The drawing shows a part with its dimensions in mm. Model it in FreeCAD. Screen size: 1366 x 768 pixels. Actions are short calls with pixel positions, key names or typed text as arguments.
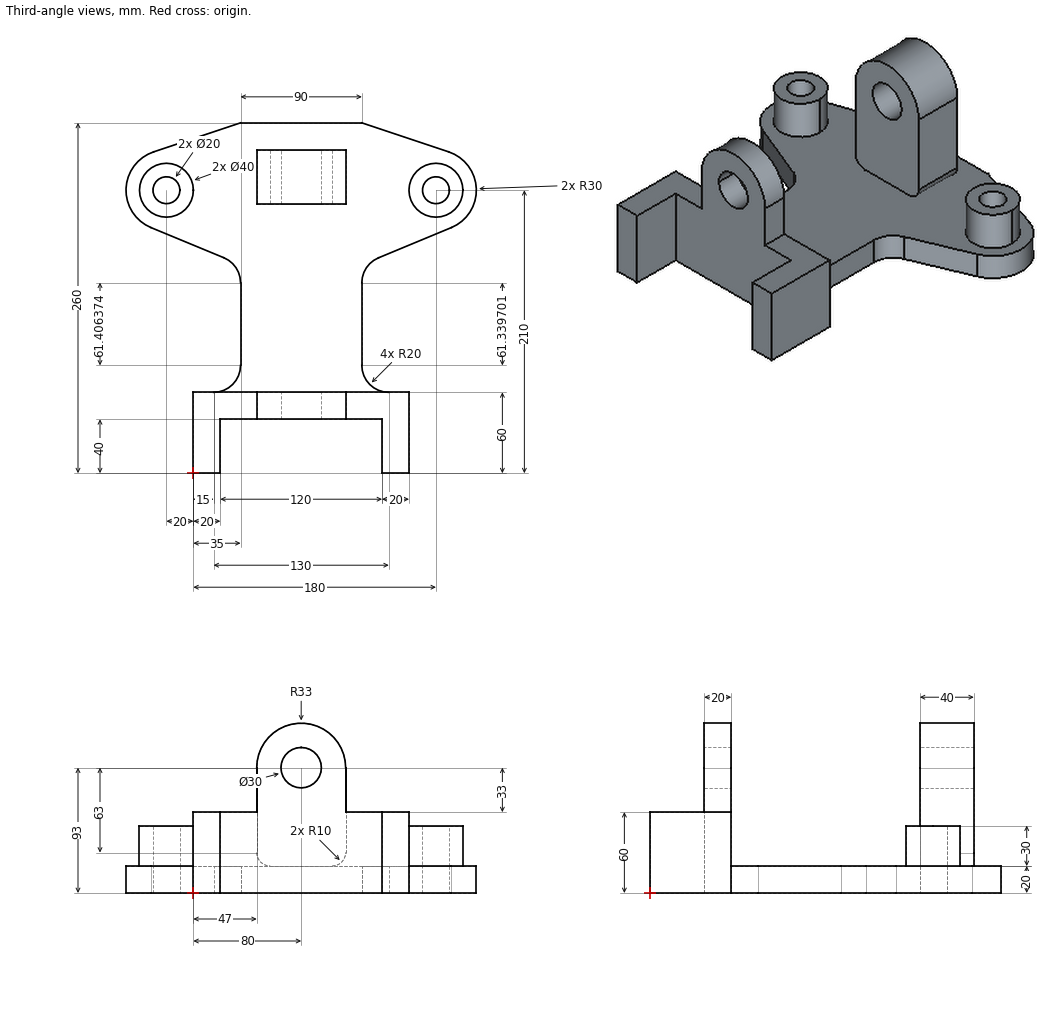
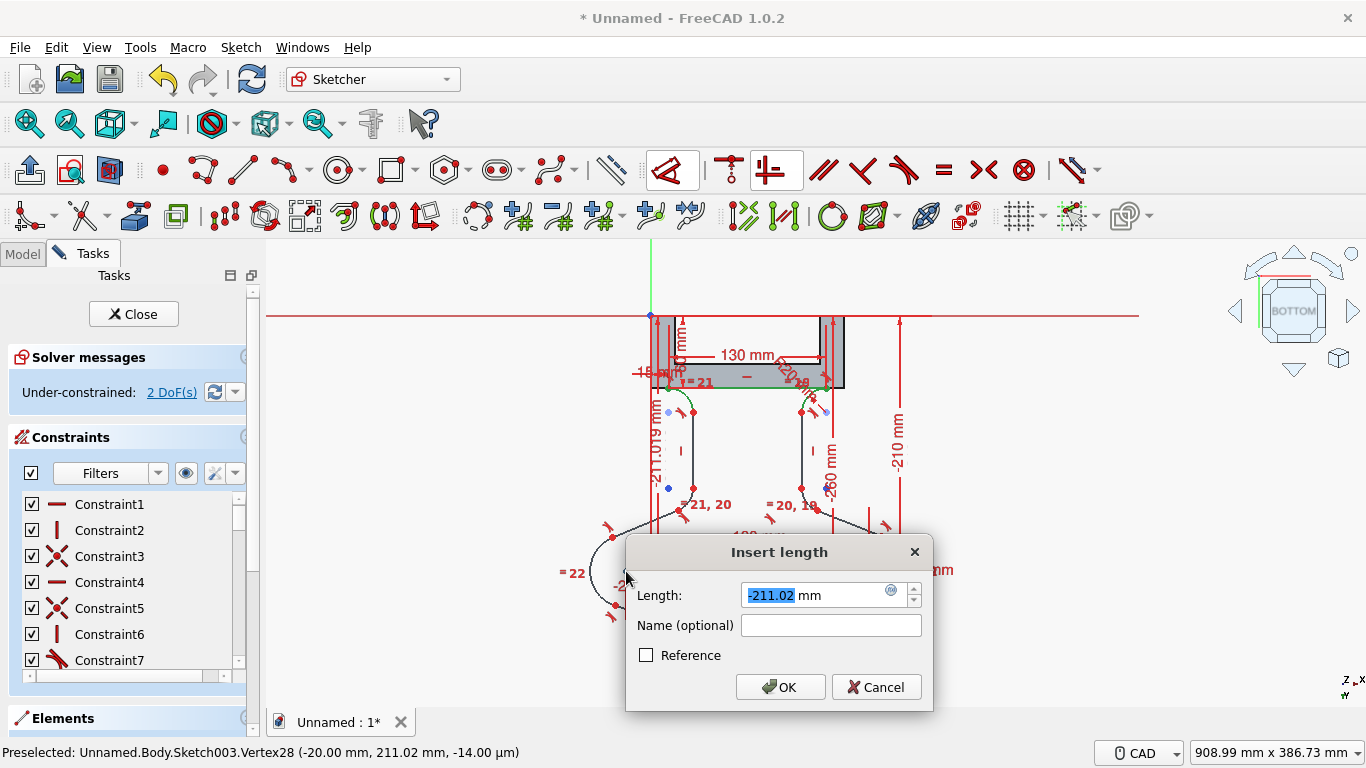
text(-210)
key(Return)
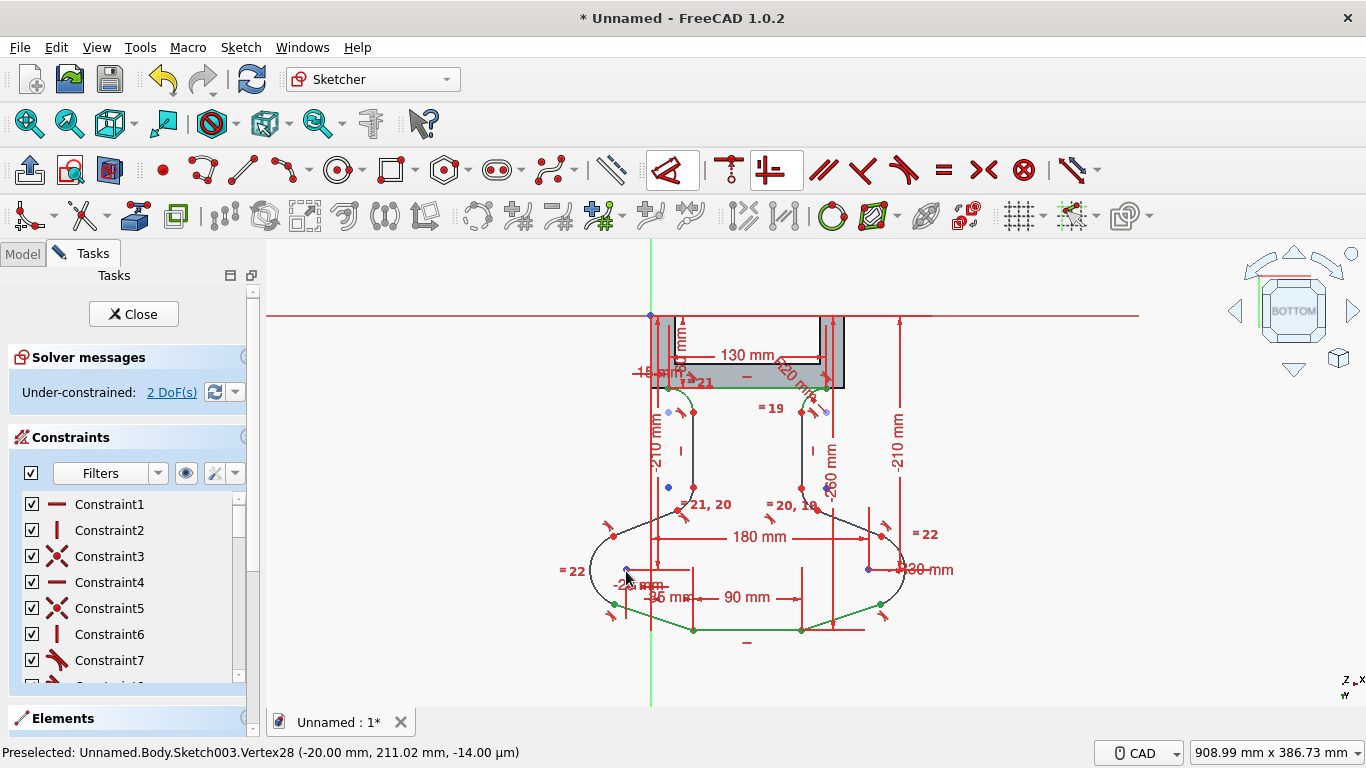
click(802, 435)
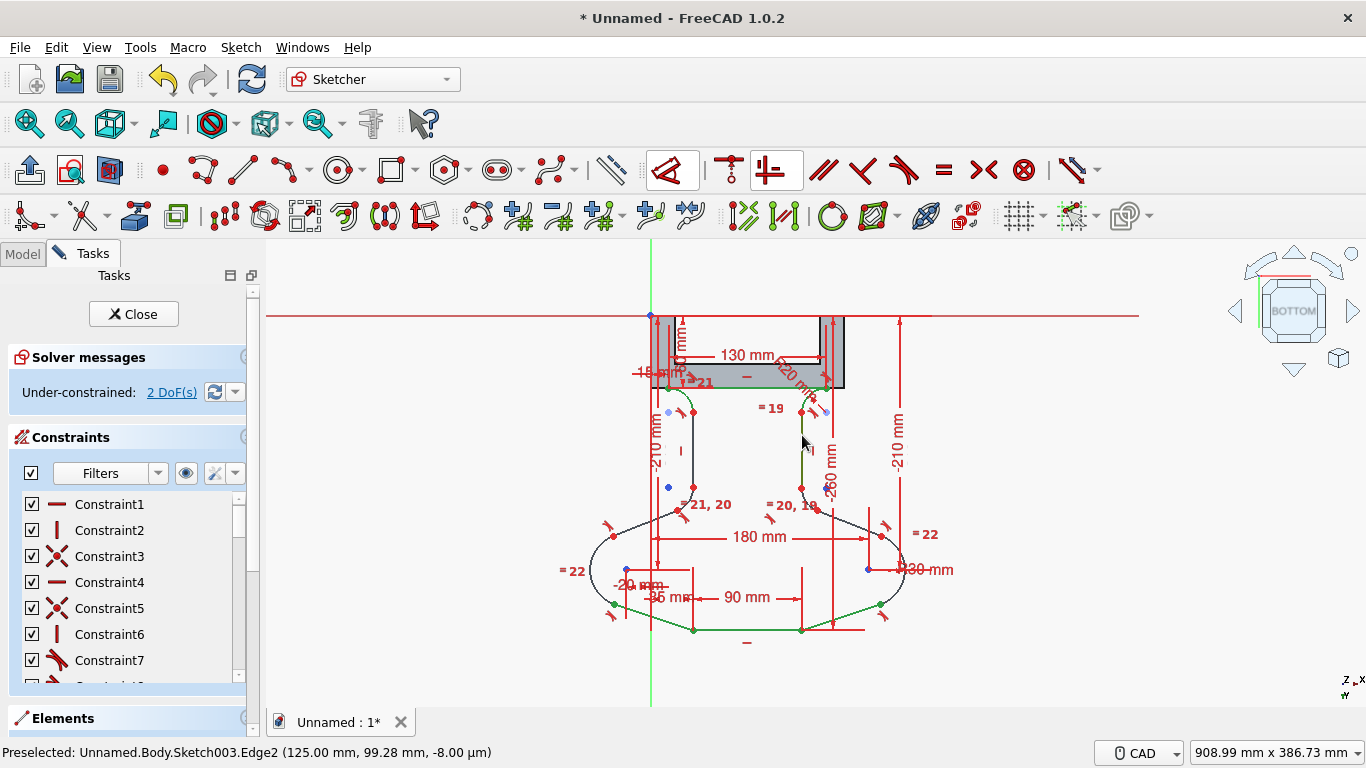
key(i)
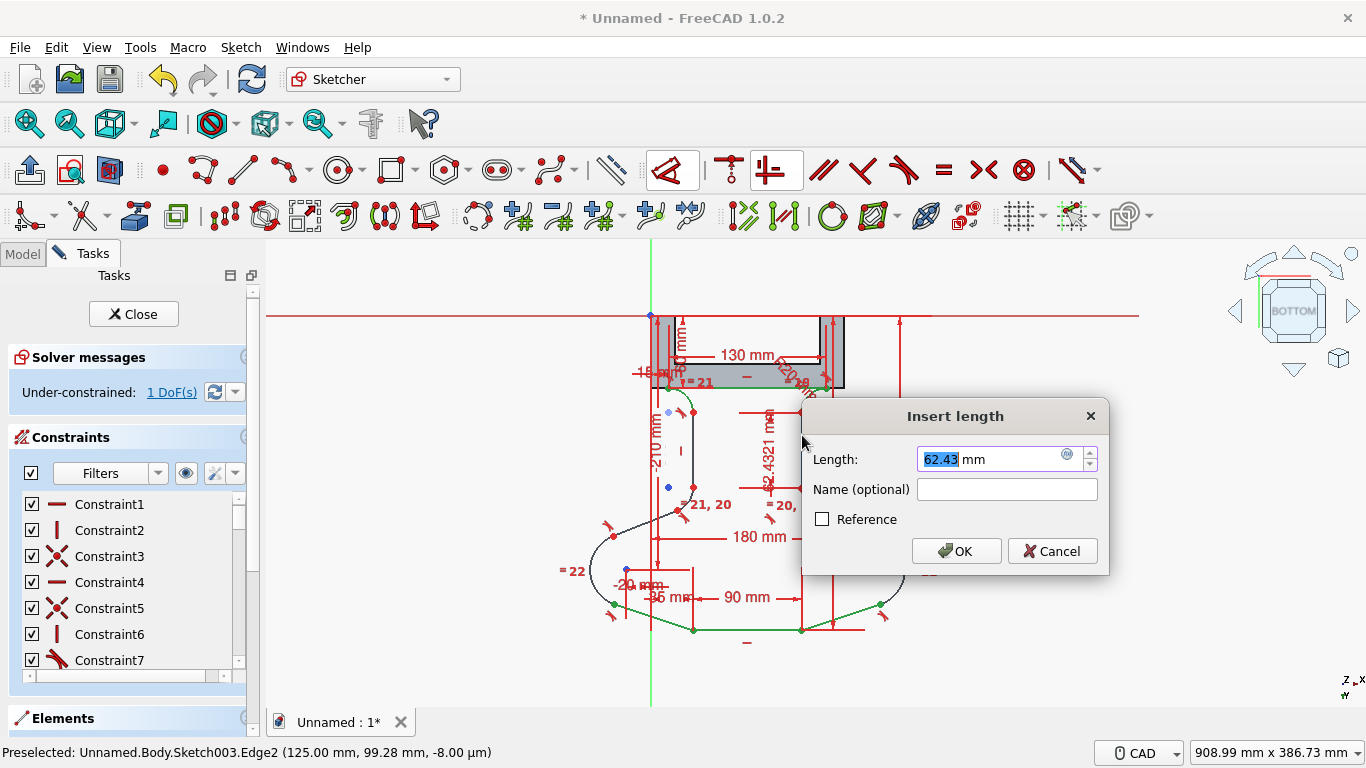
text(61.339701)
key(Return)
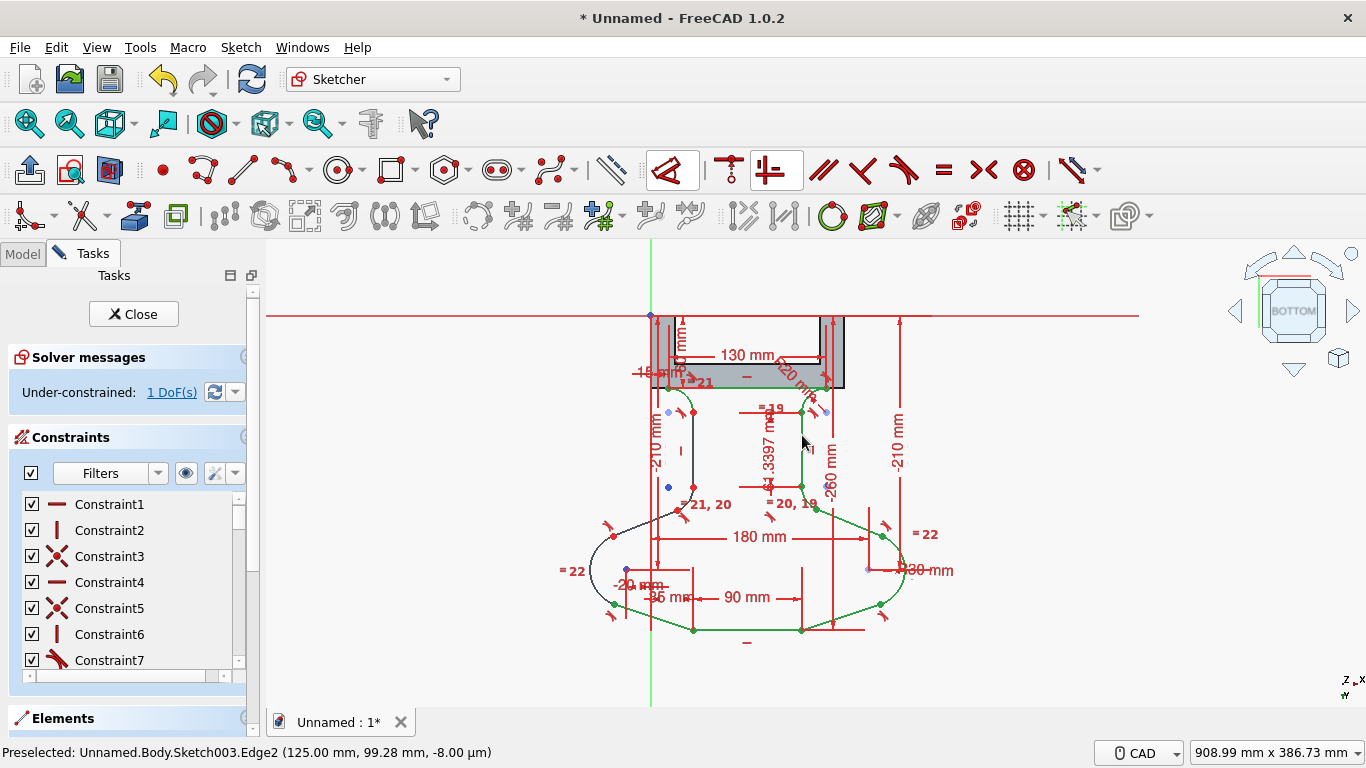
click(693, 465)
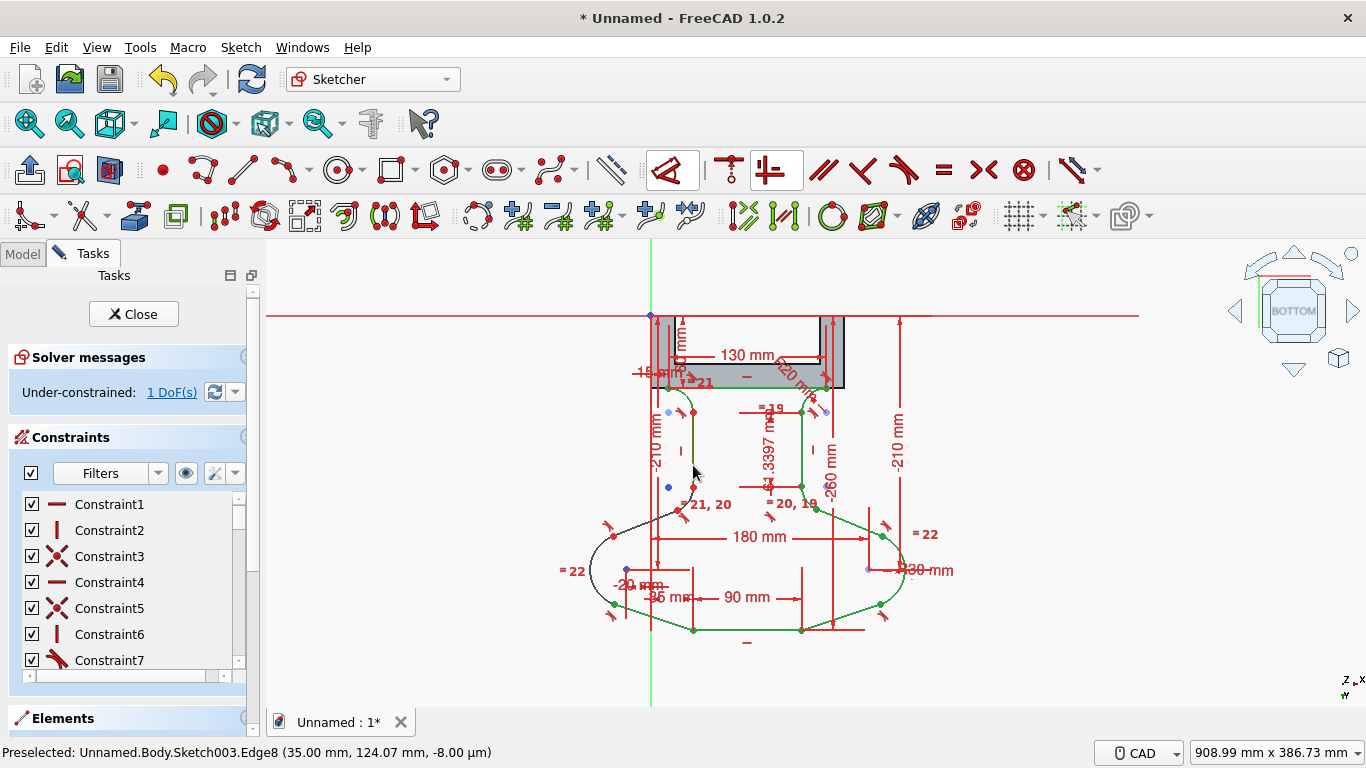
key(i)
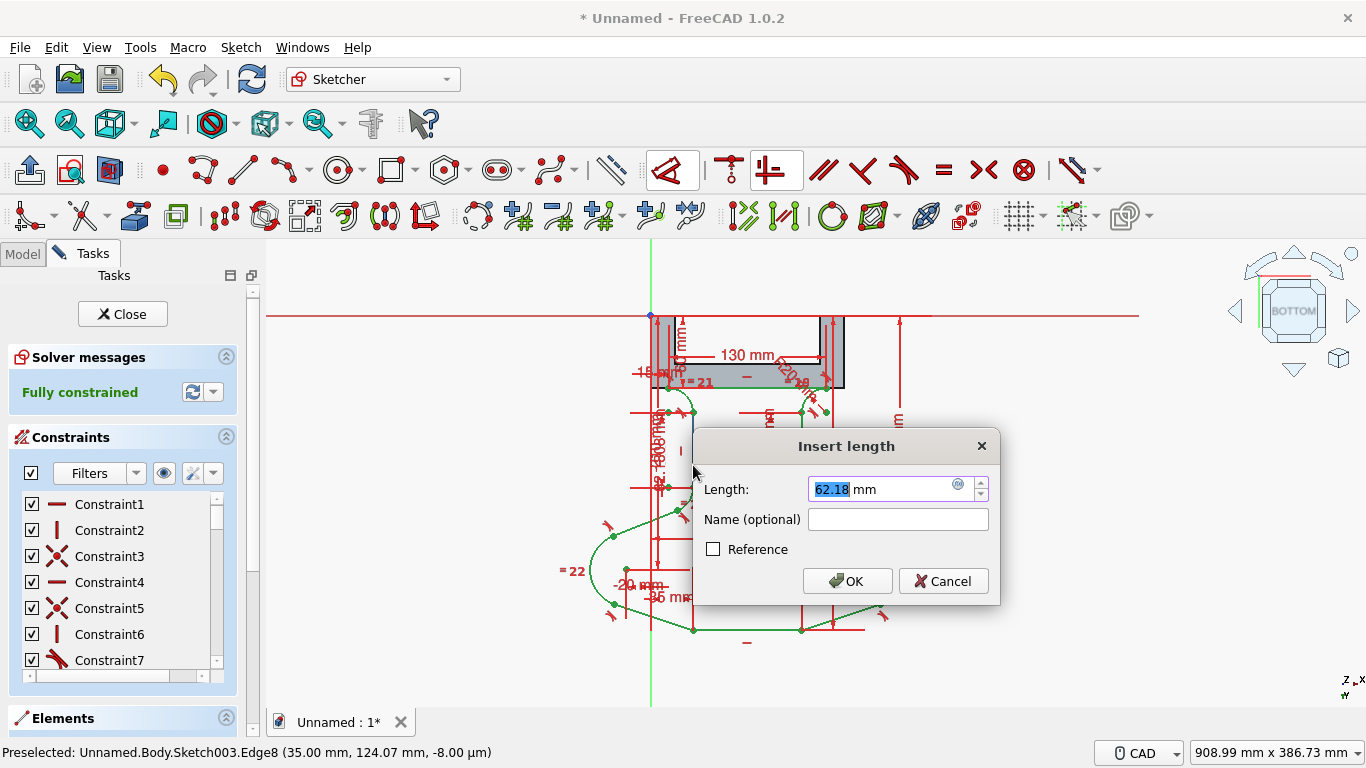
text(61.406374)
key(Return)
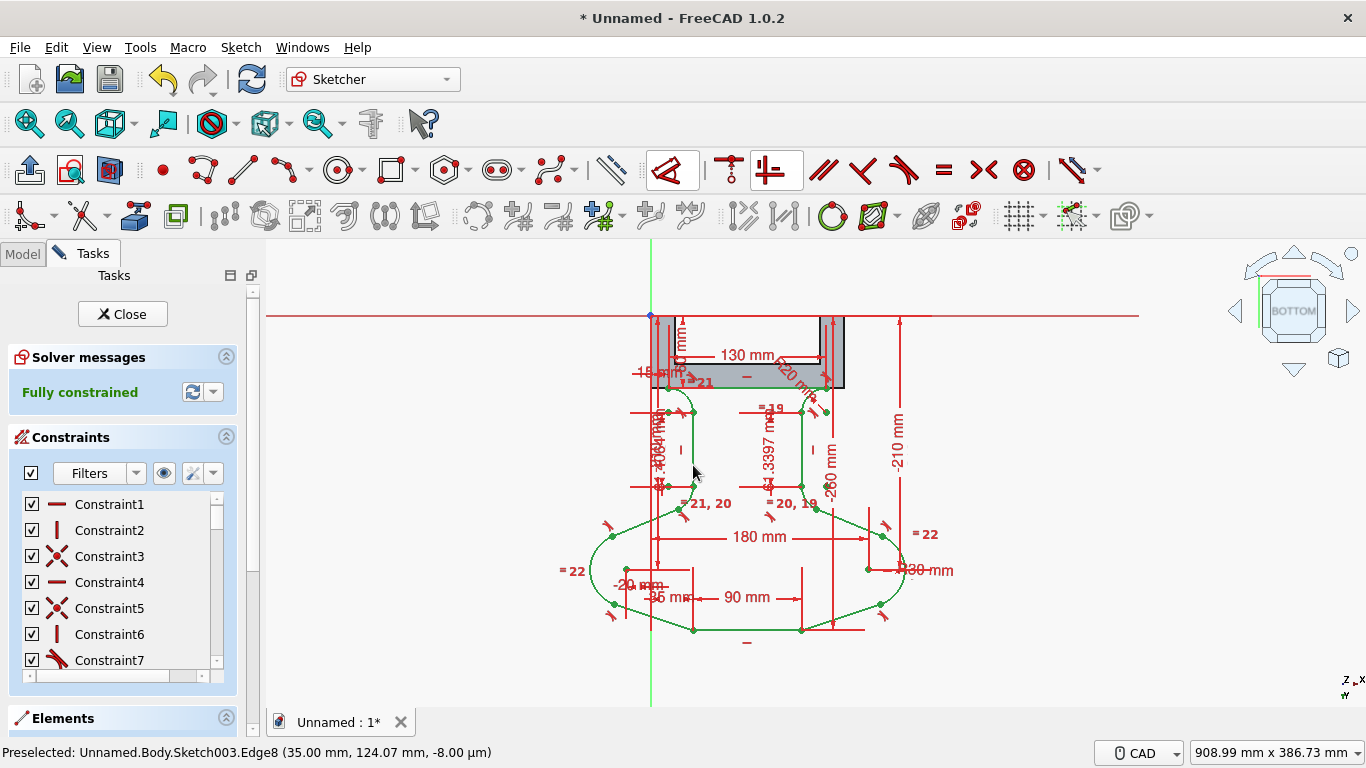
click(123, 314)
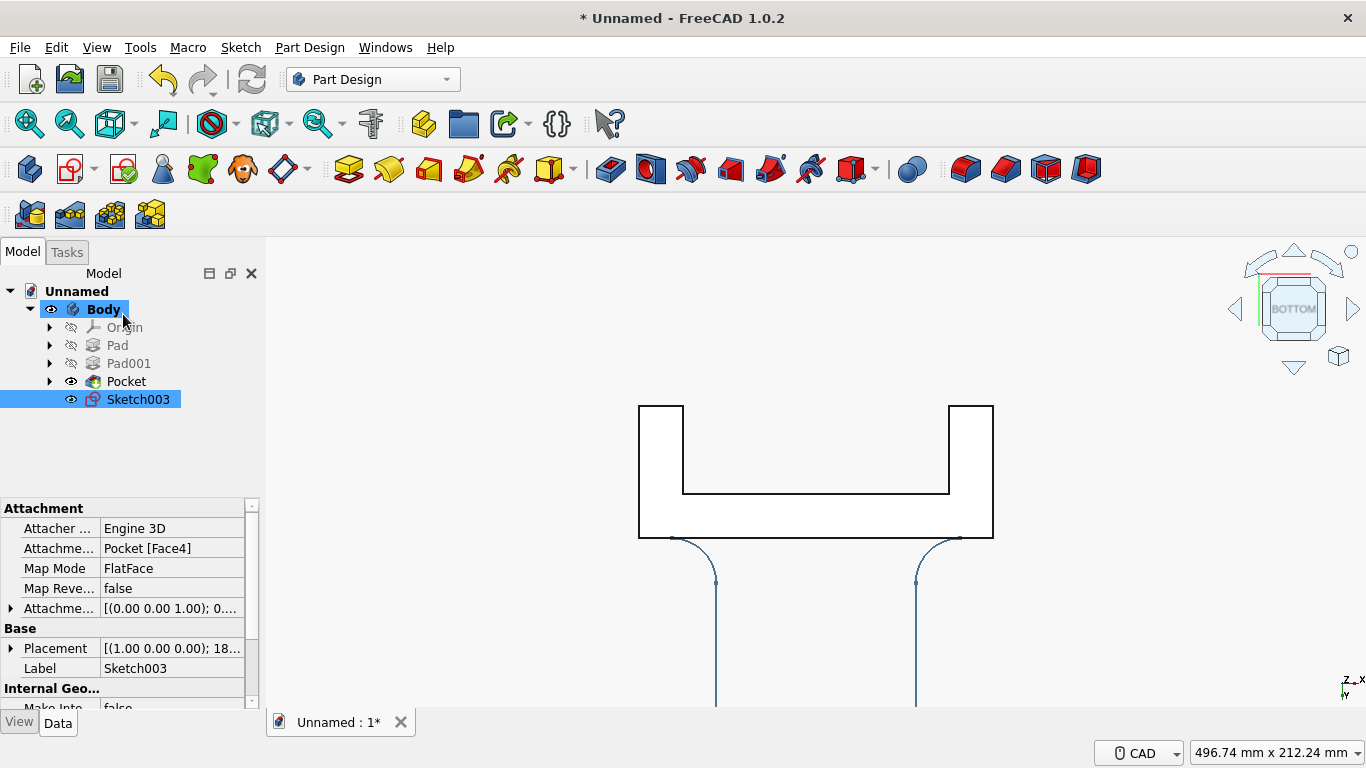
click(350, 170)